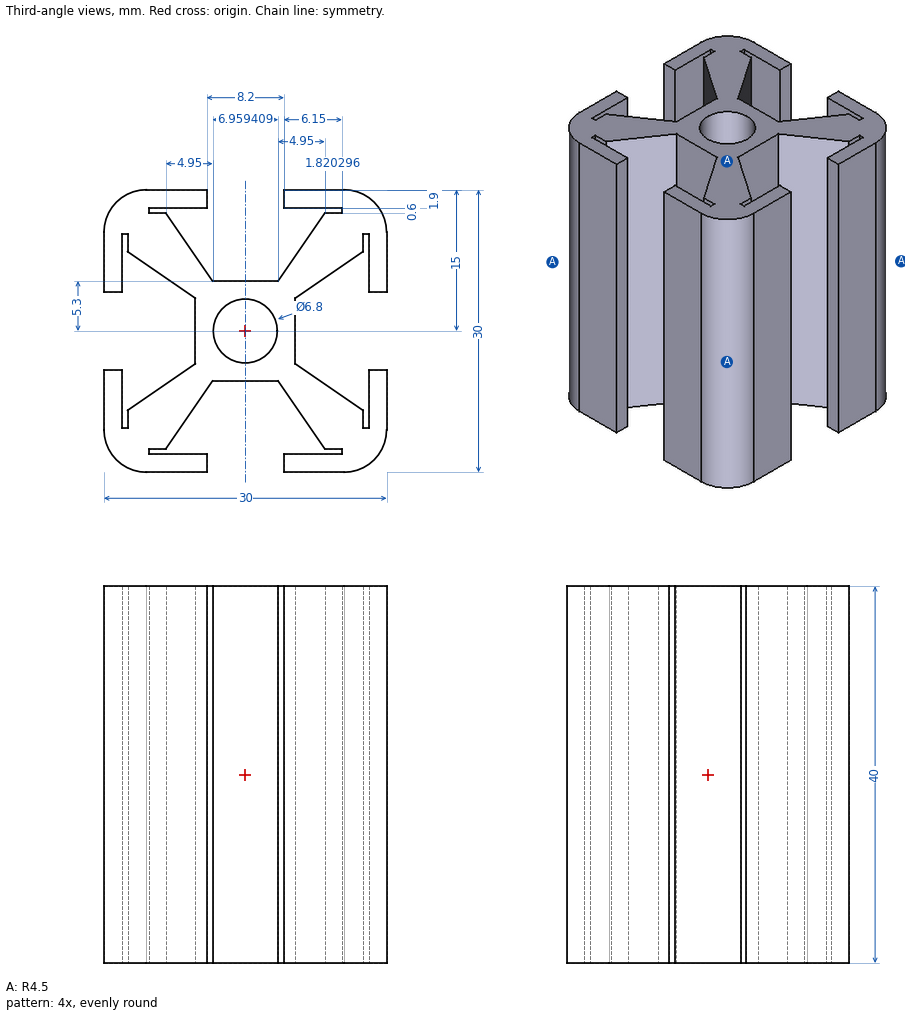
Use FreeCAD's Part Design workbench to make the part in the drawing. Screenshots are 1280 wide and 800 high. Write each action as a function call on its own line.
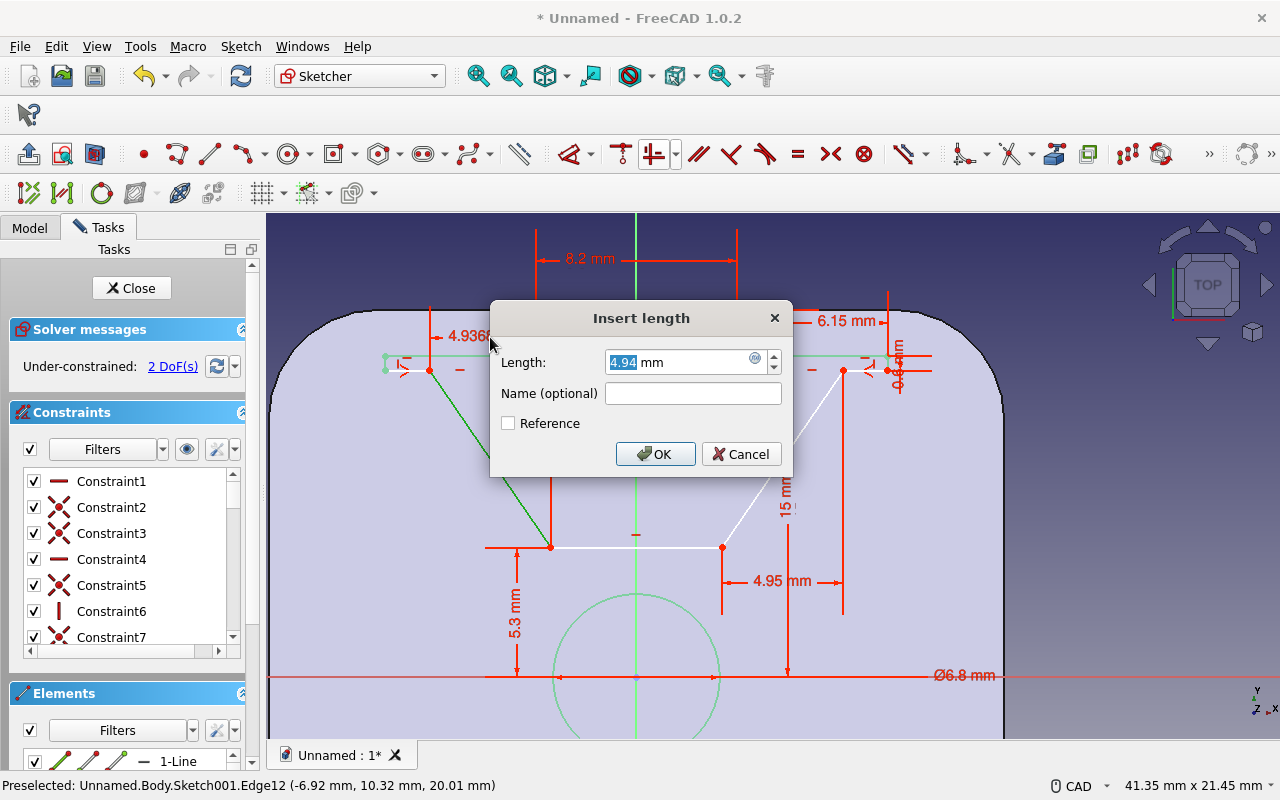
text(4.95)
key(Return)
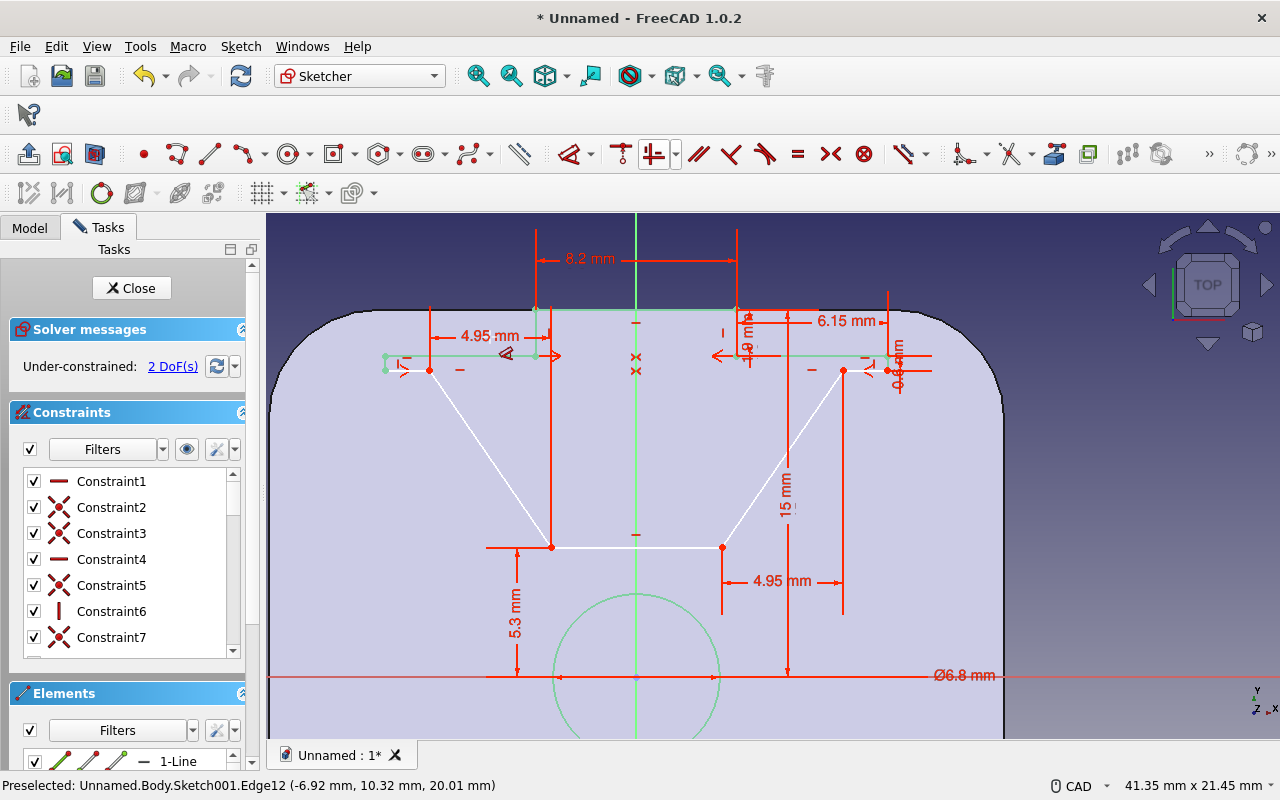
click(603, 548)
click(597, 582)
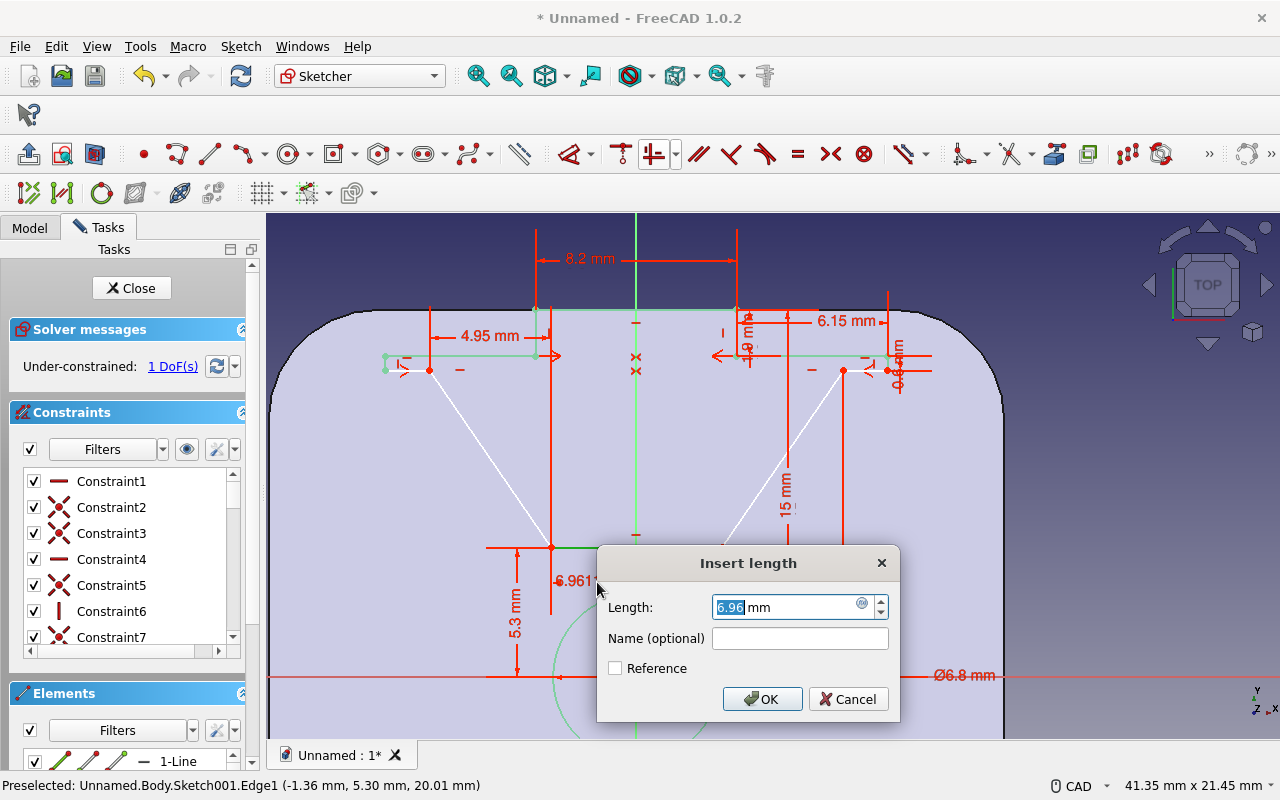
text(6.959409)
key(Return)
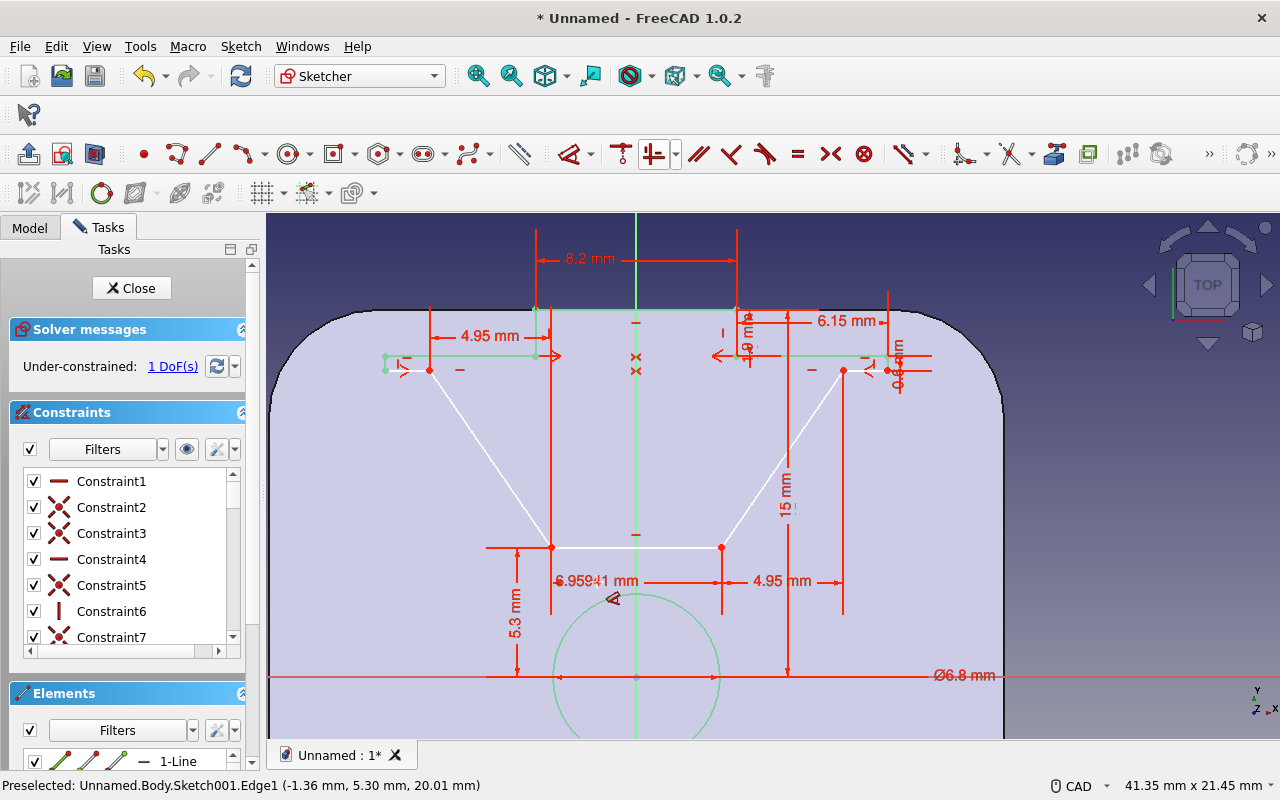
click(857, 371)
click(866, 405)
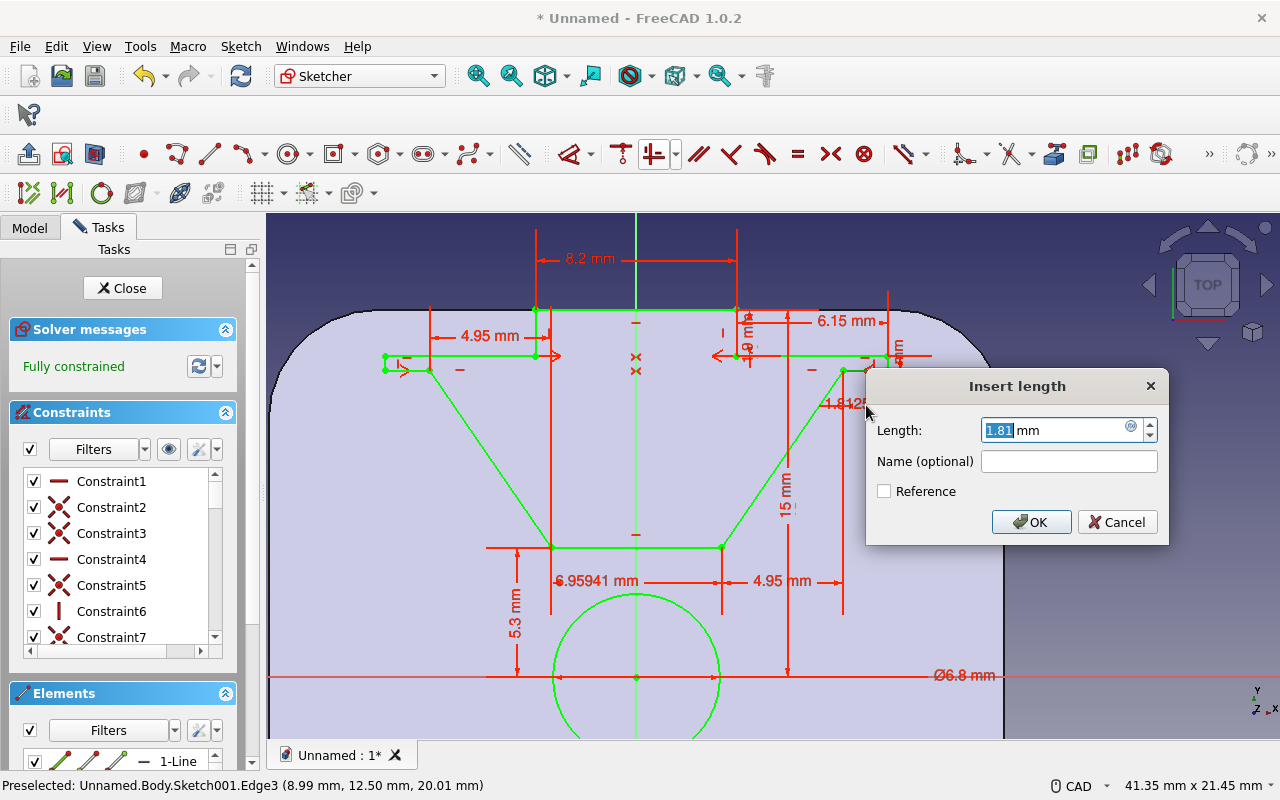
text(1.820296)
key(Return)
key(Escape)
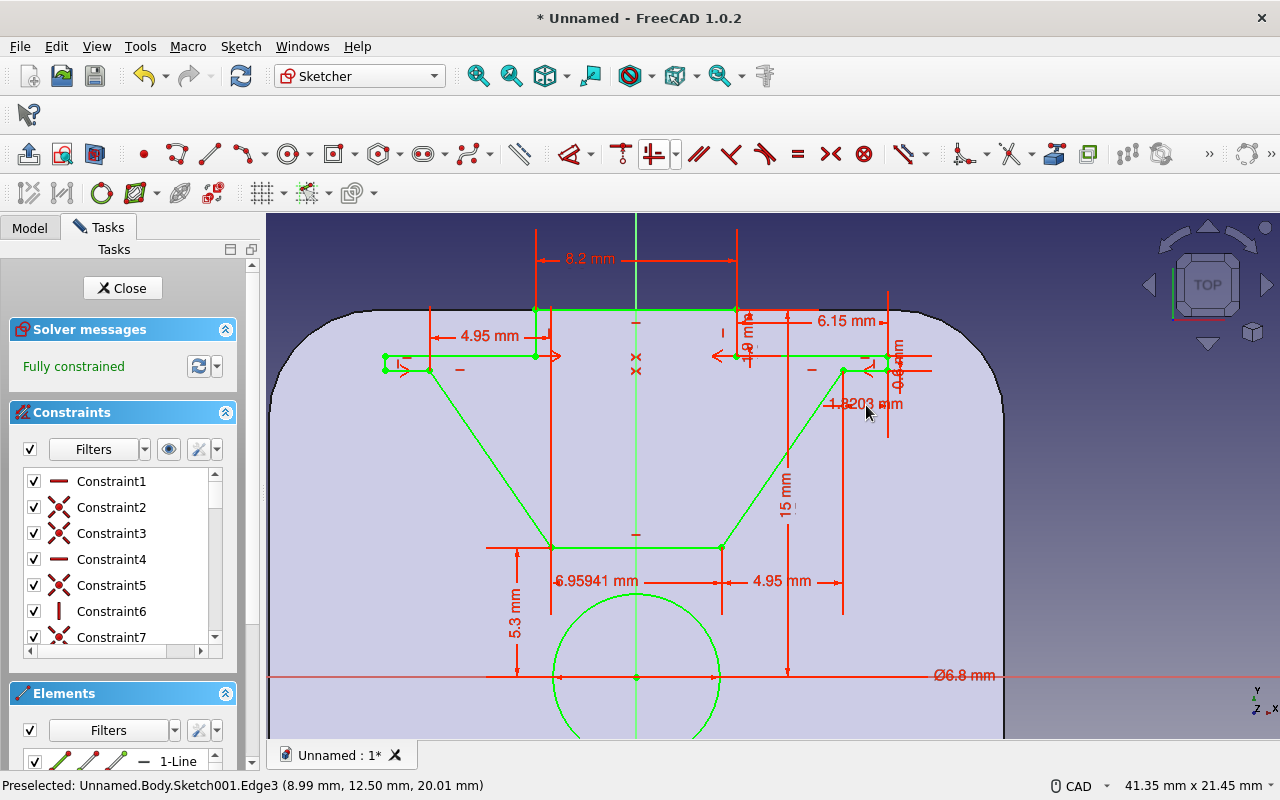
click(123, 288)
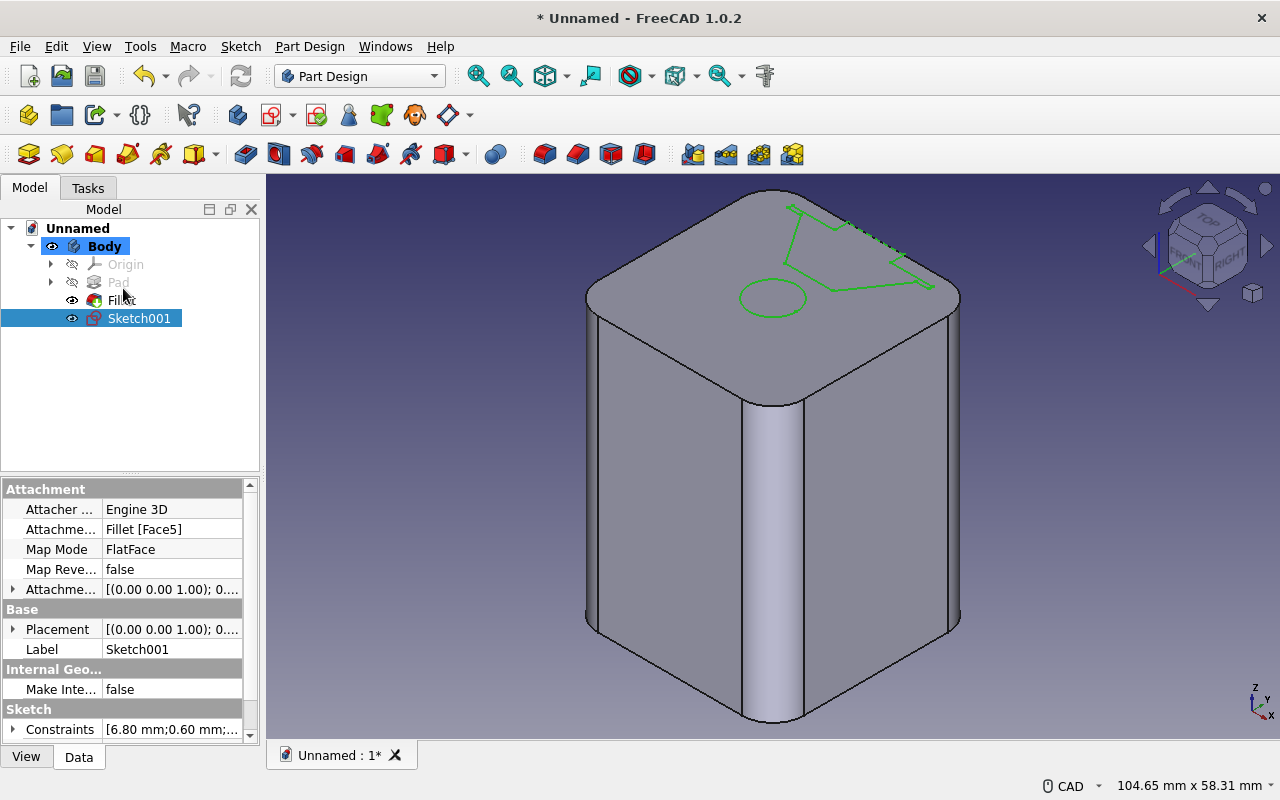
click(246, 154)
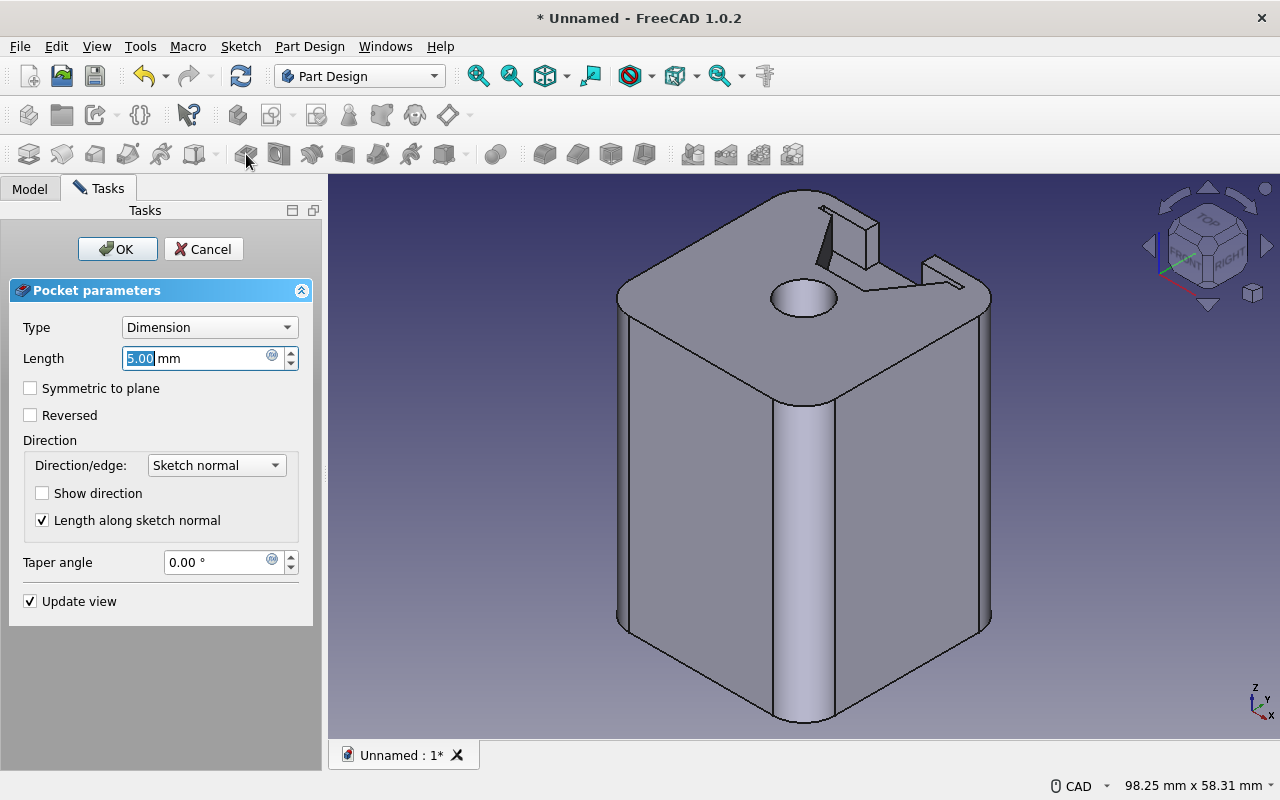
click(210, 328)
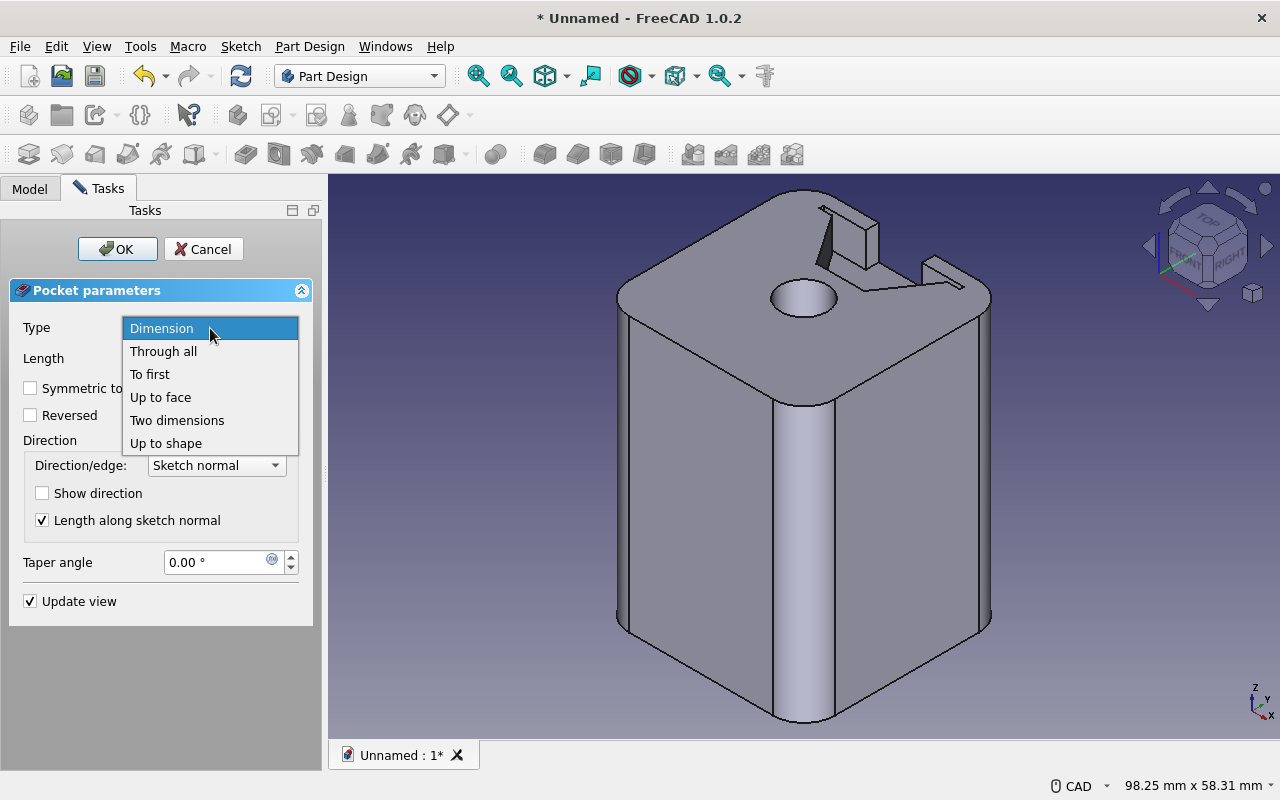
click(208, 352)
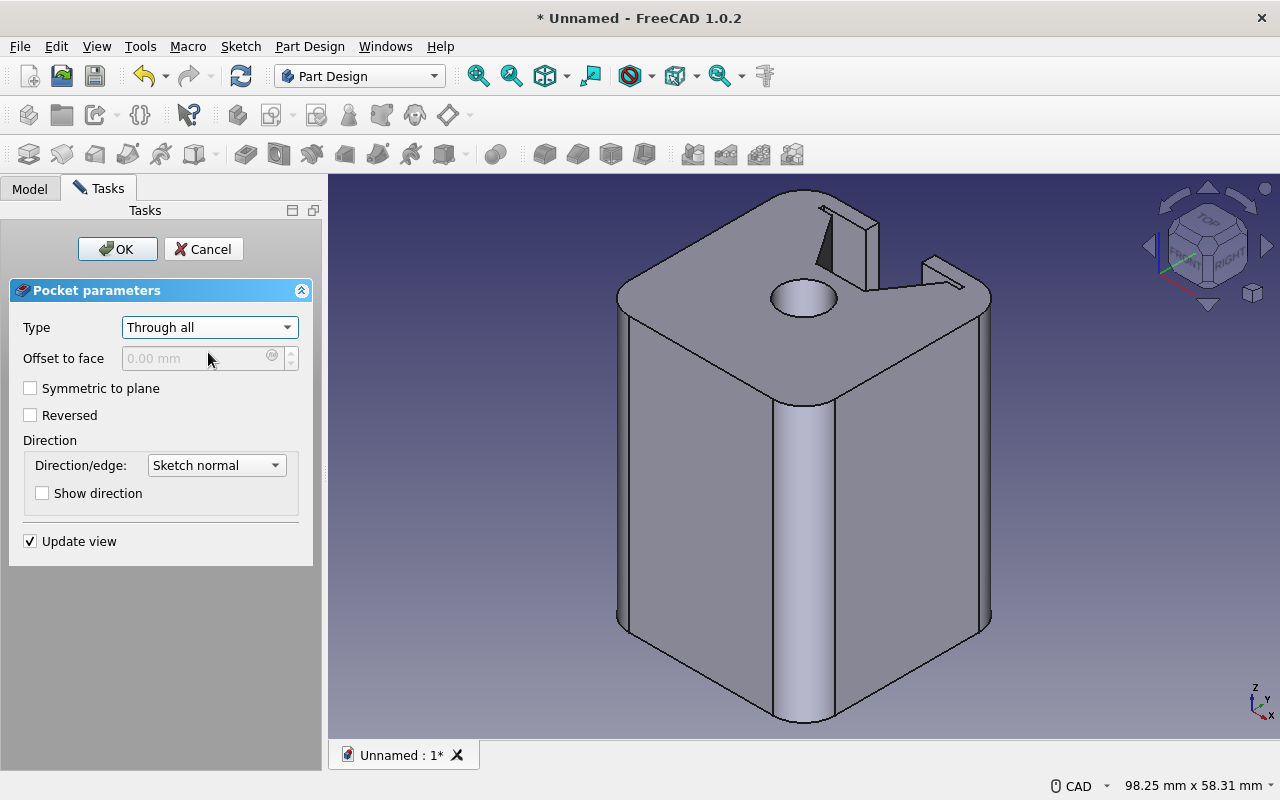
click(118, 249)